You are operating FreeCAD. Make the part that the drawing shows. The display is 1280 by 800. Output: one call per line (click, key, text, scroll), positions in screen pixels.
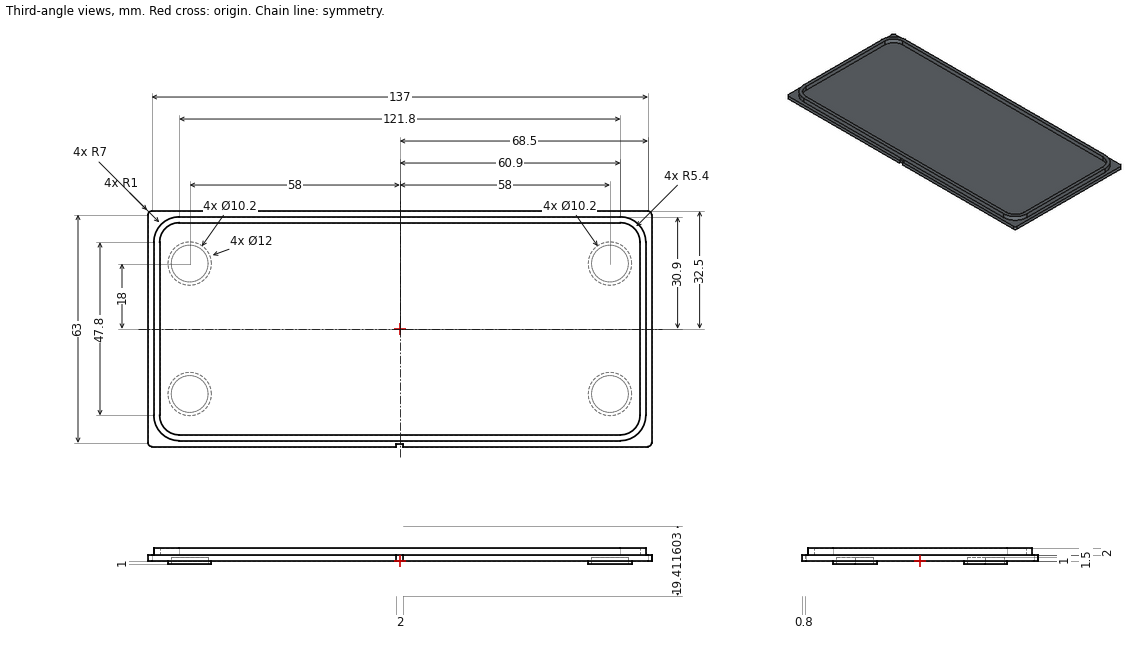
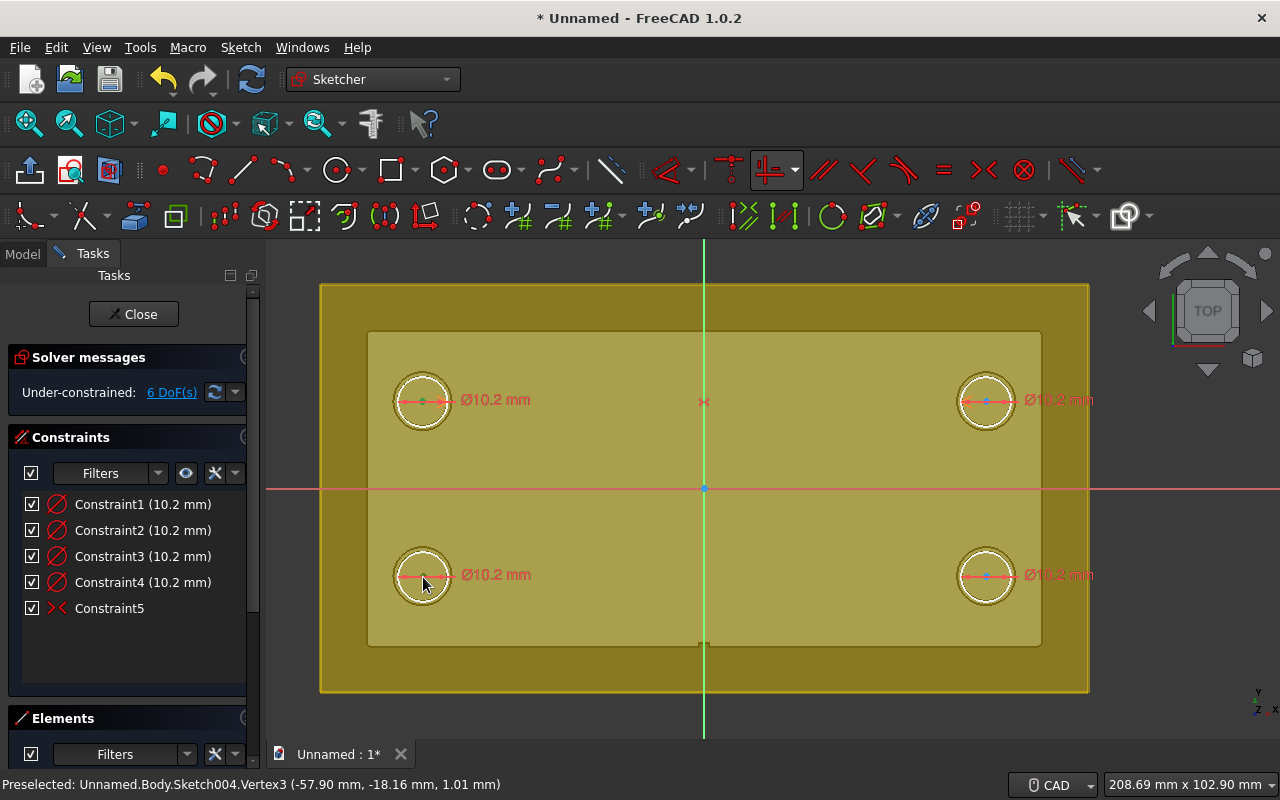
click(353, 489)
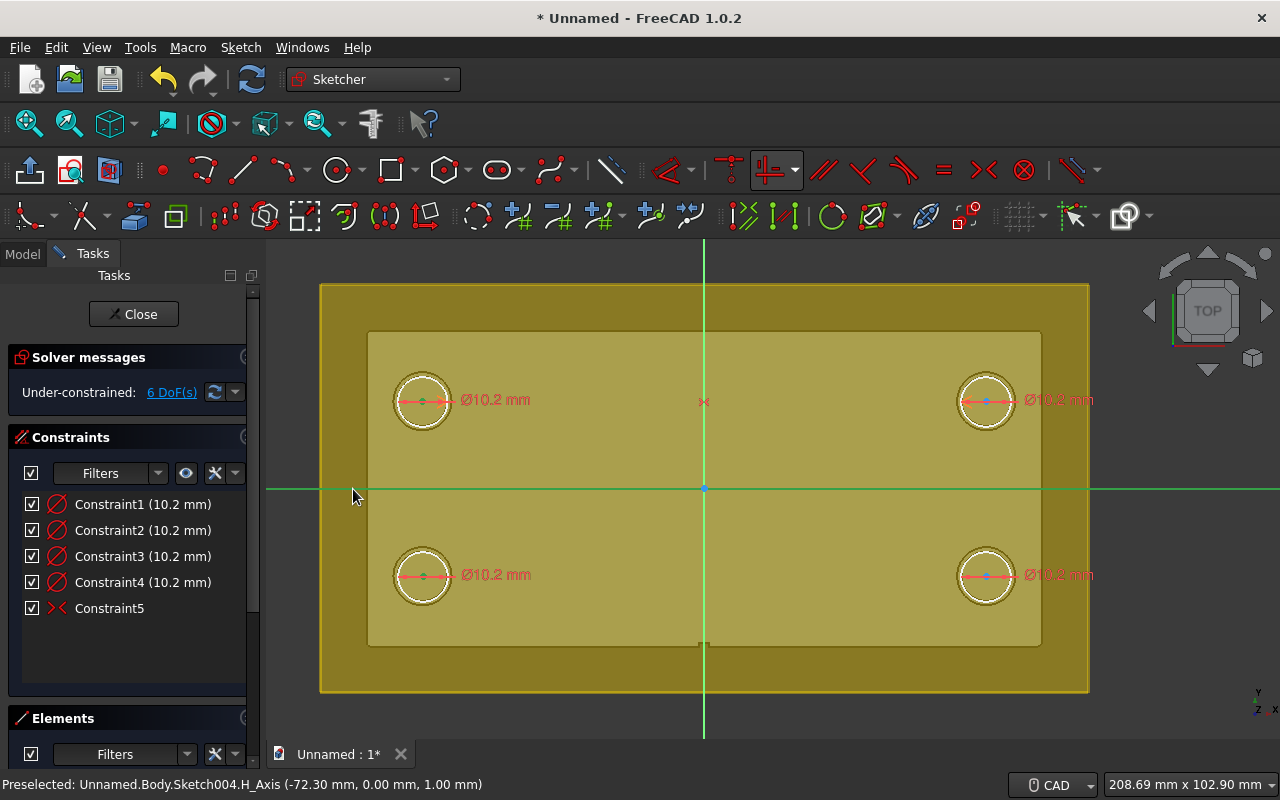
click(984, 170)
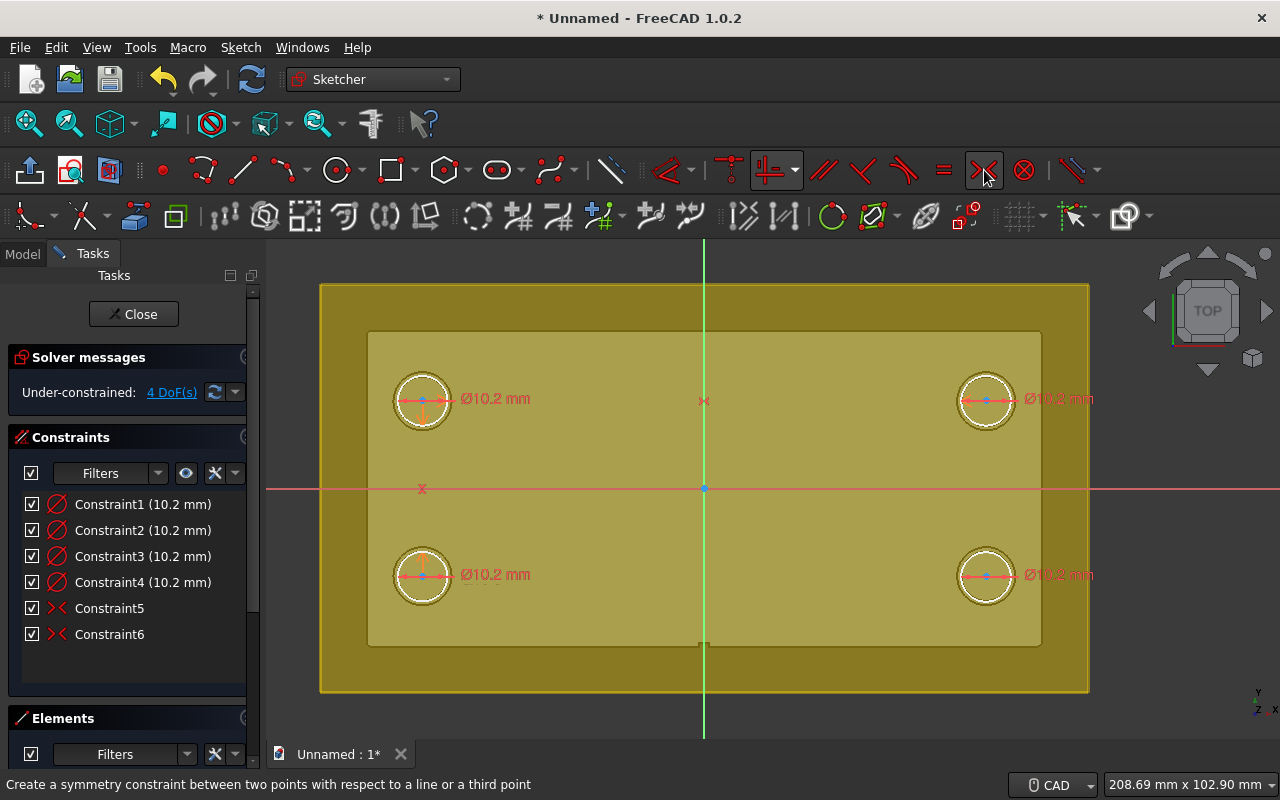
click(986, 401)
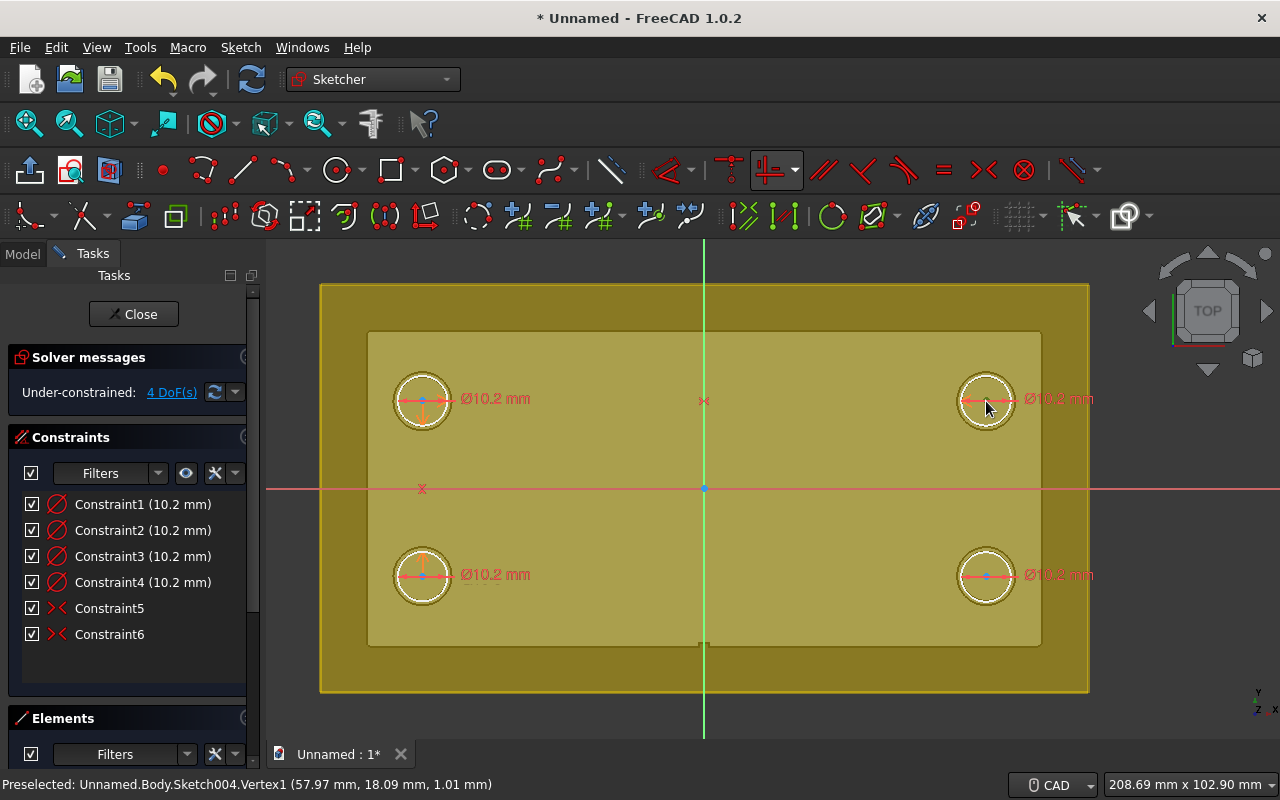
click(986, 577)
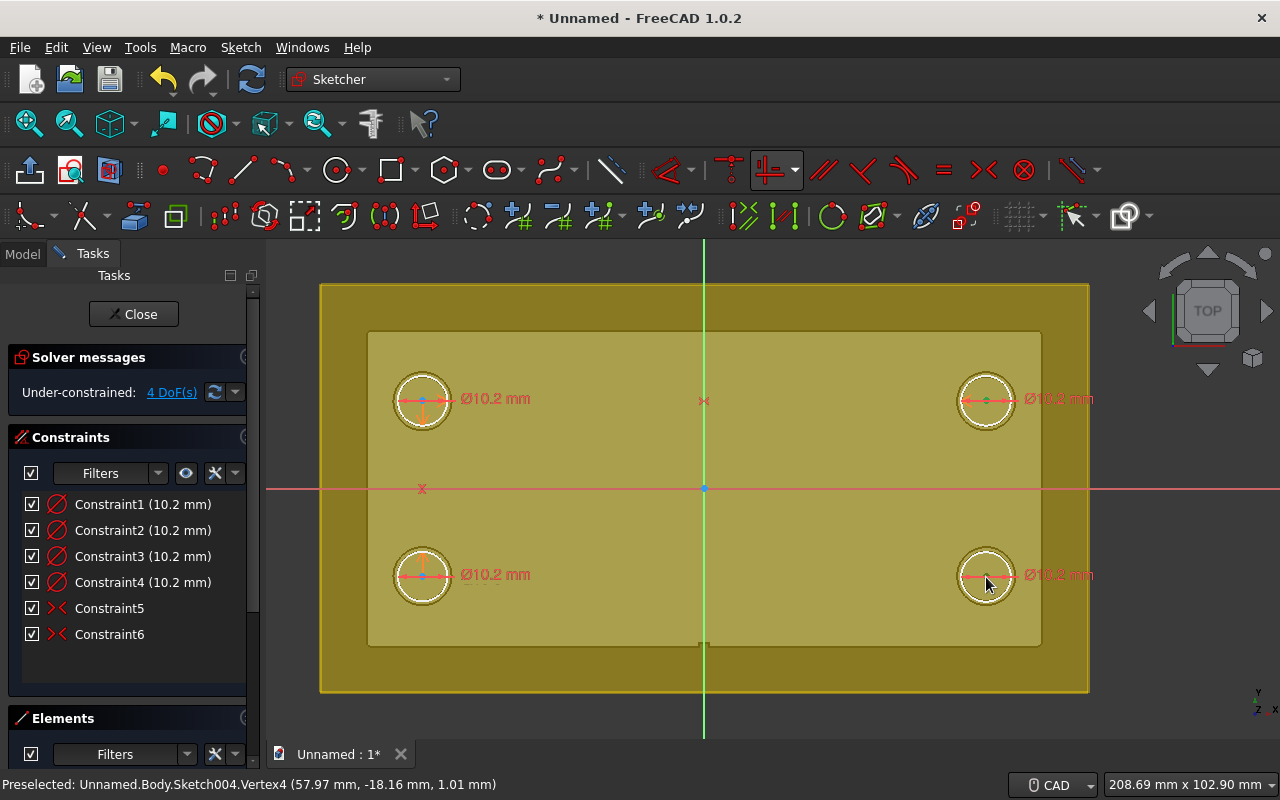
click(353, 489)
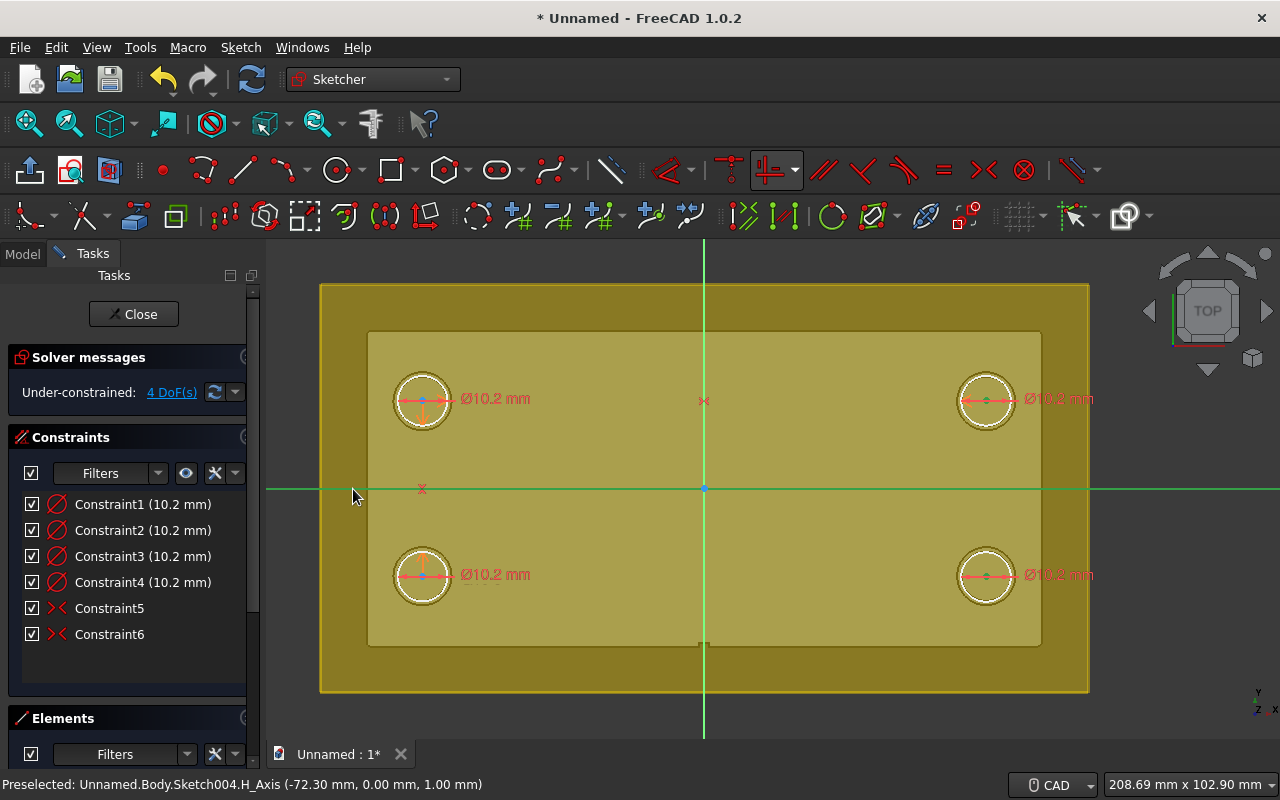
click(984, 170)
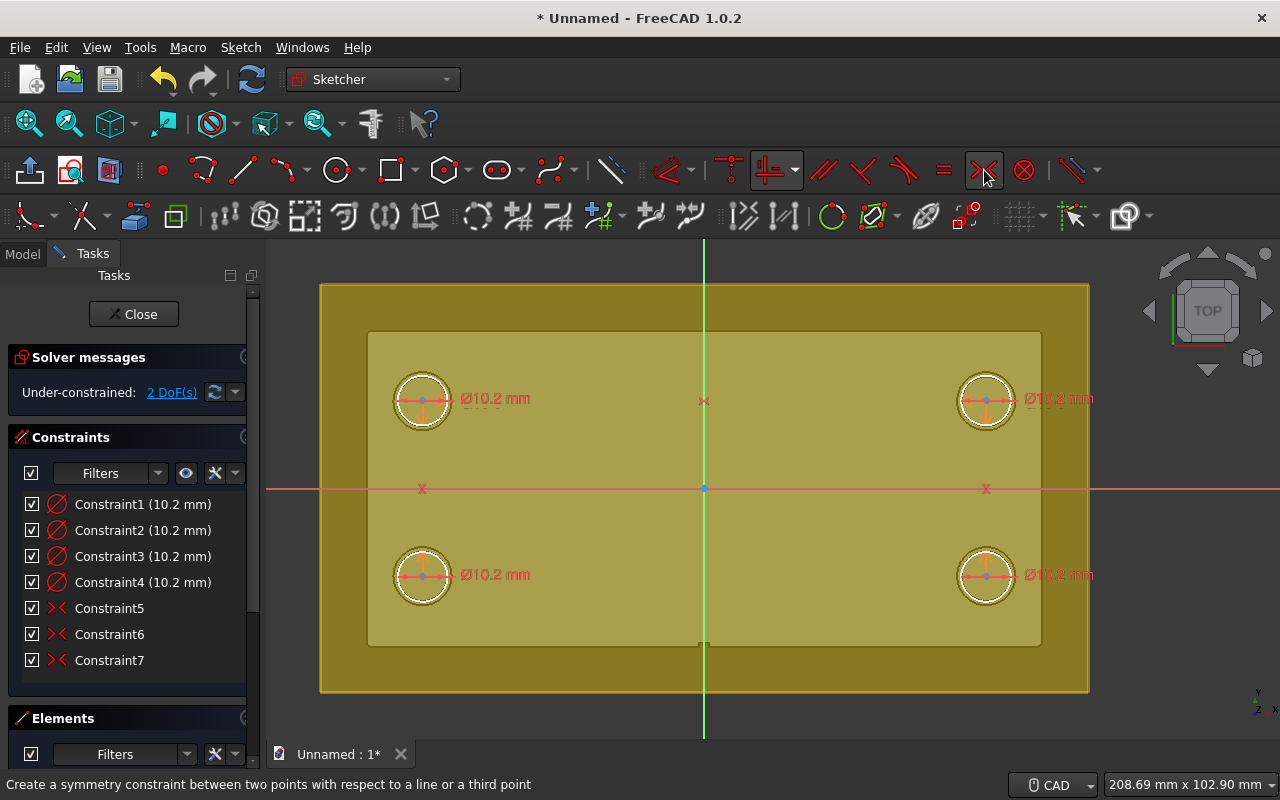
click(666, 170)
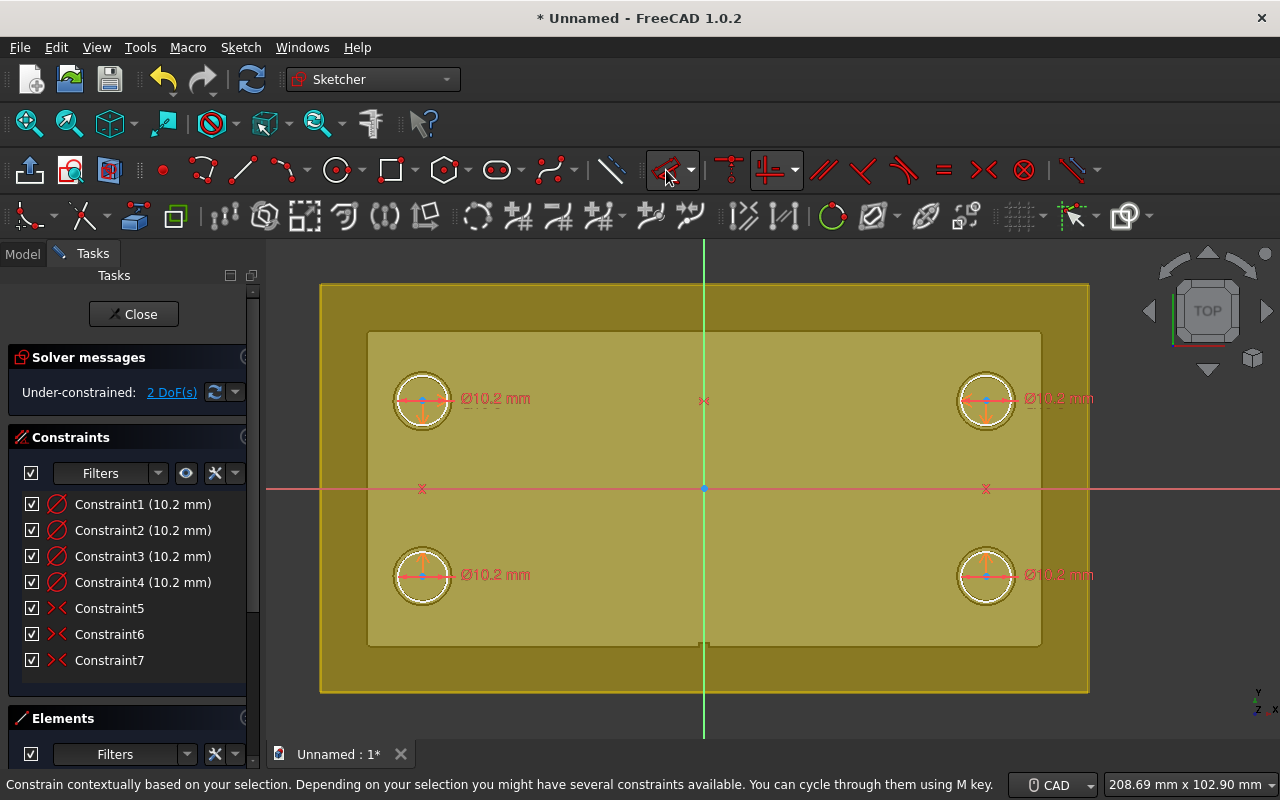
click(986, 401)
click(845, 367)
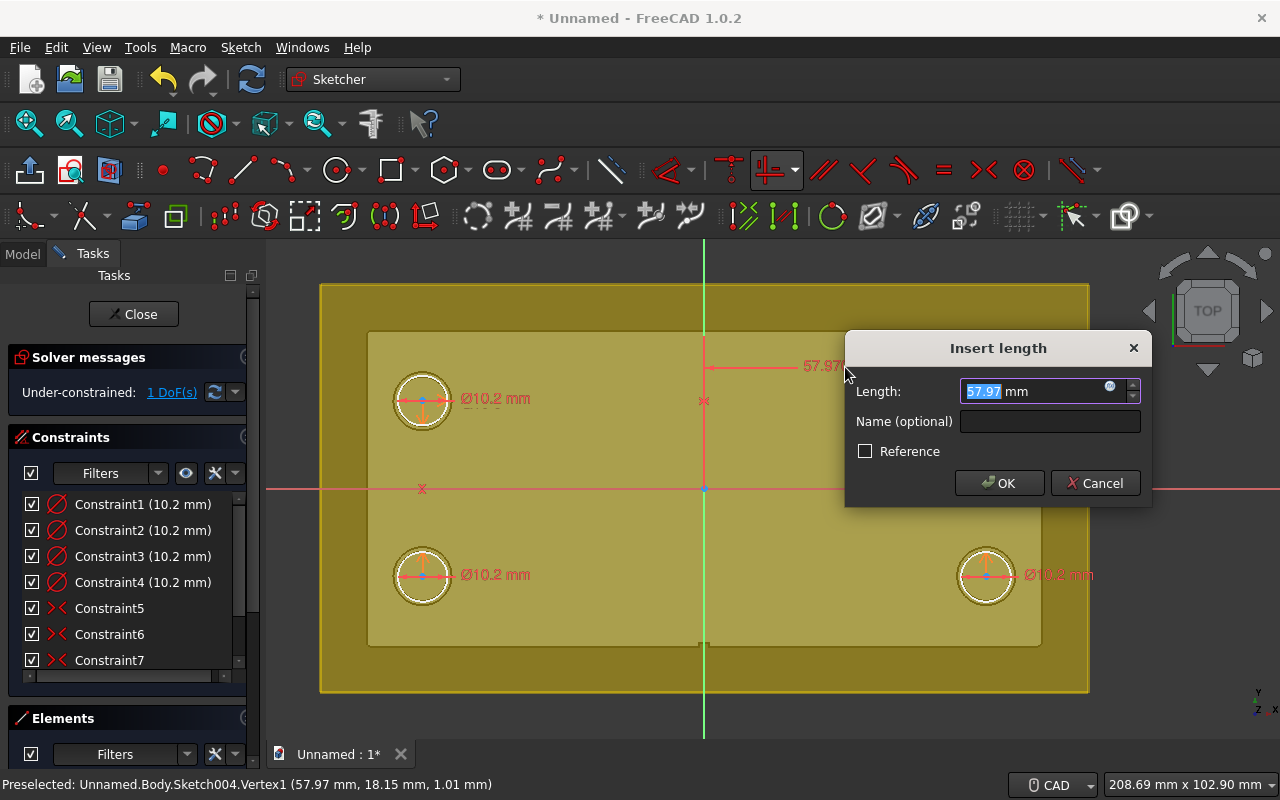
text(58)
key(Return)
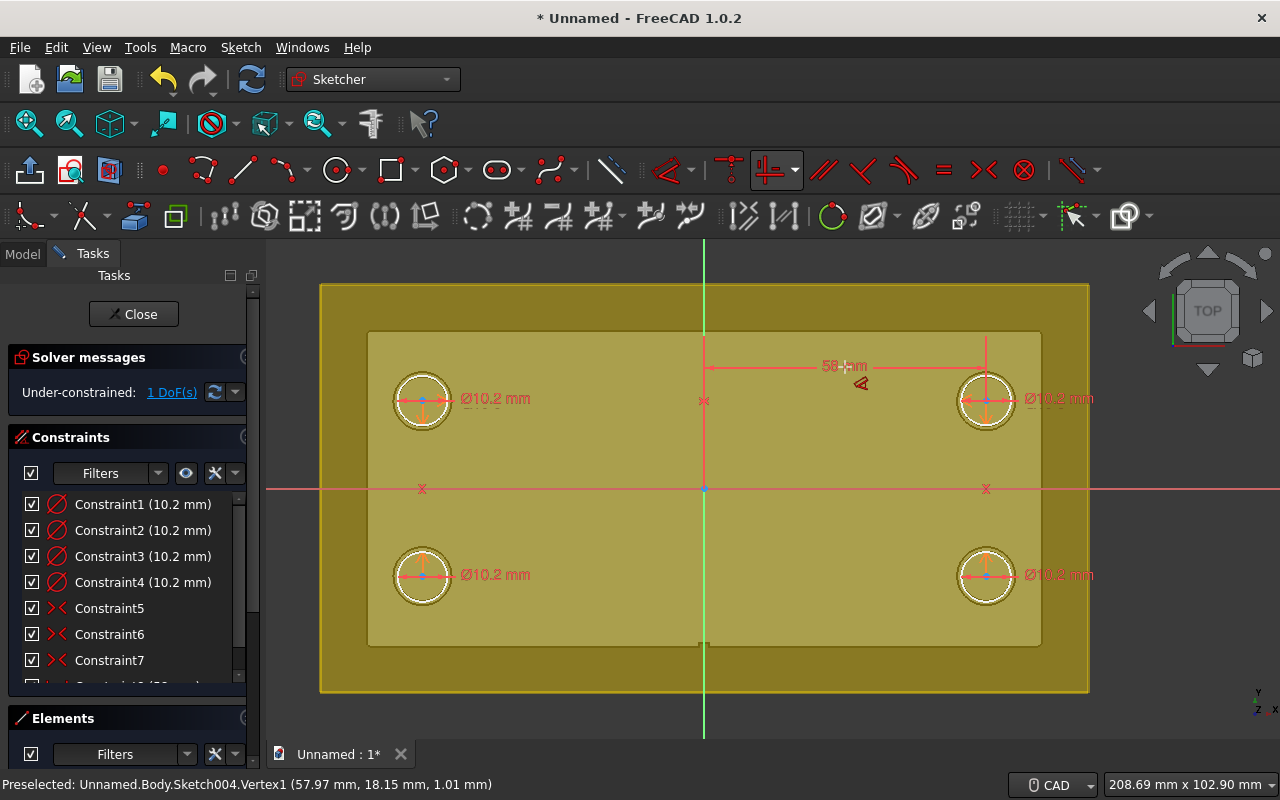
click(986, 401)
click(1020, 445)